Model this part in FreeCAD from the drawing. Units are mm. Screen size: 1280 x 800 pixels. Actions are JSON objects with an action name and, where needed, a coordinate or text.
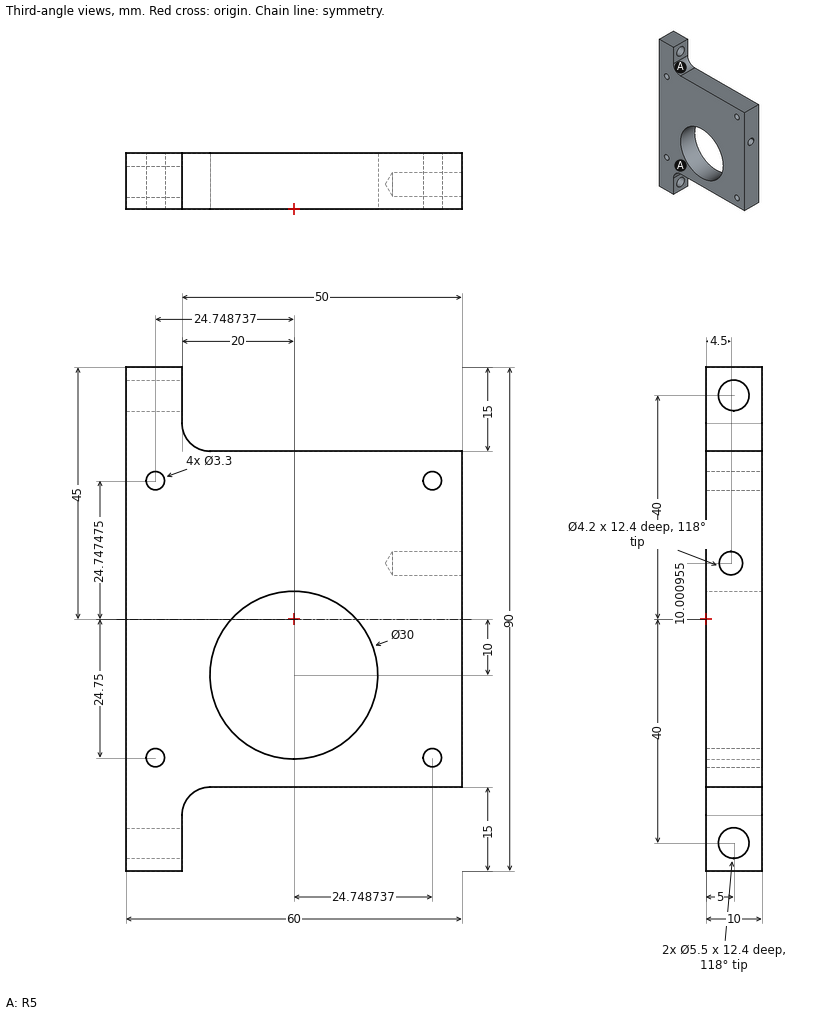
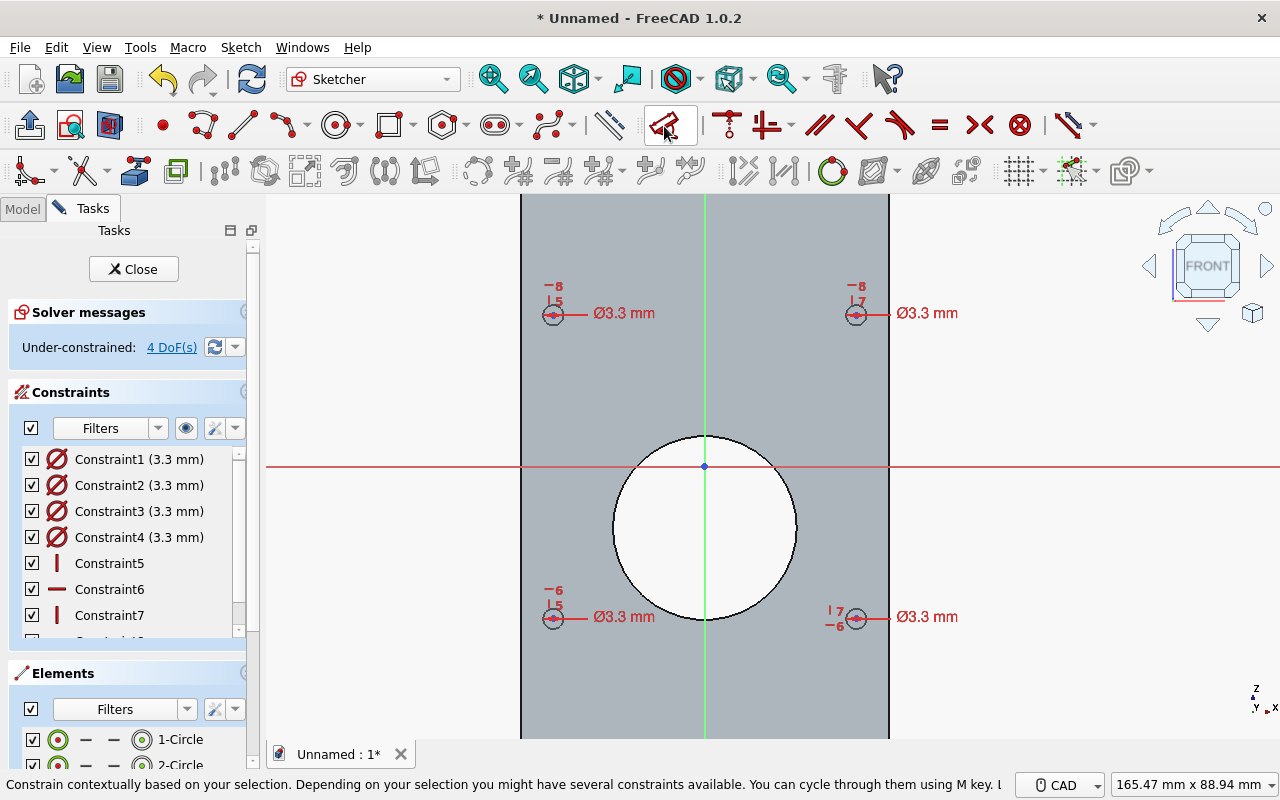
{"action": "left_click", "coordinate": [553, 619]}
{"action": "left_click", "coordinate": [519, 543]}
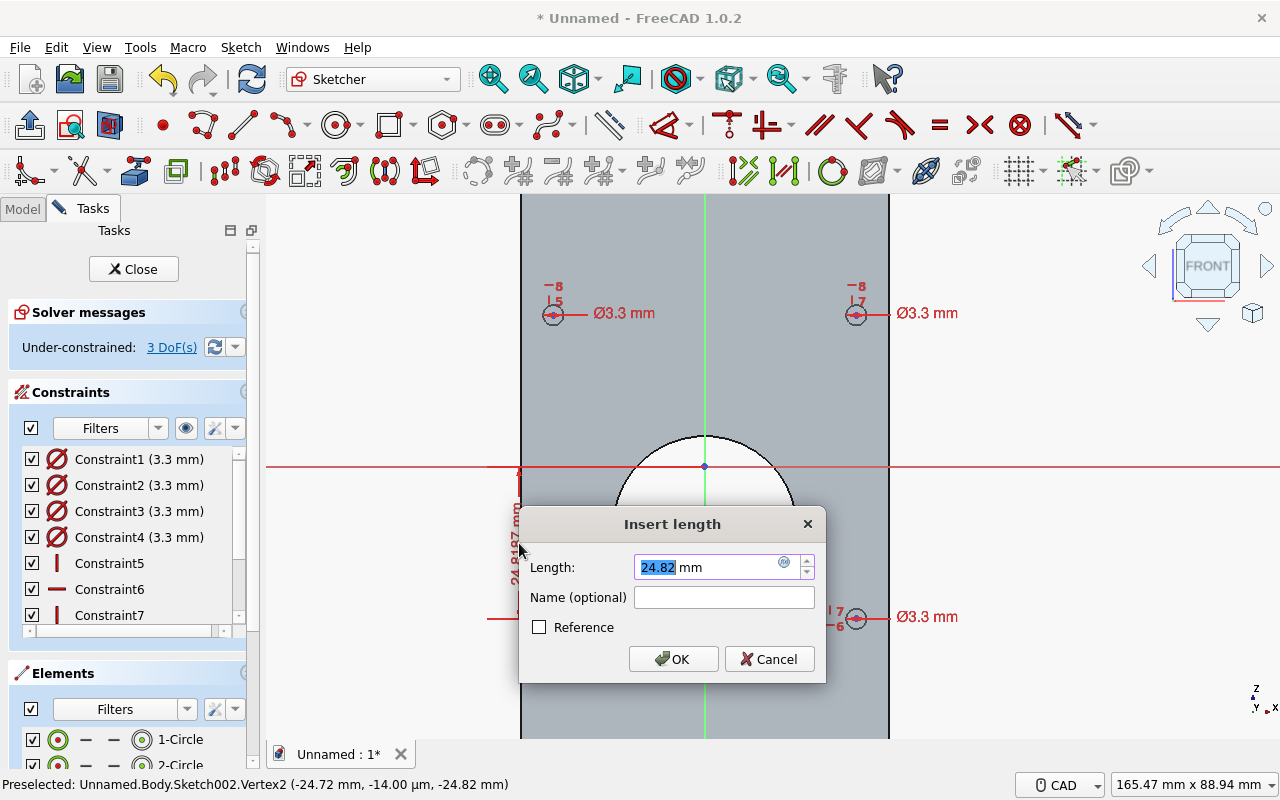
{"action": "type", "text": "24.75"}
{"action": "key", "text": "Return"}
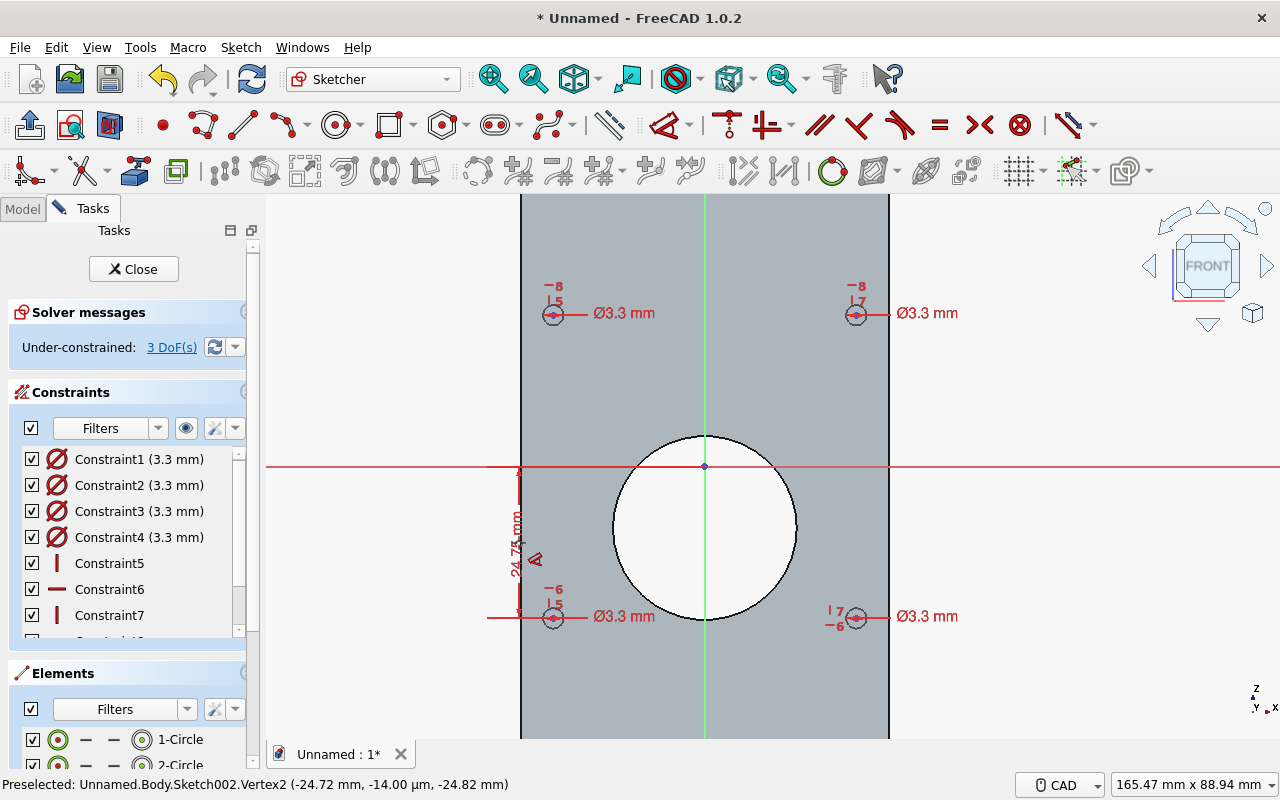
{"action": "left_click", "coordinate": [553, 315]}
{"action": "left_click", "coordinate": [629, 281]}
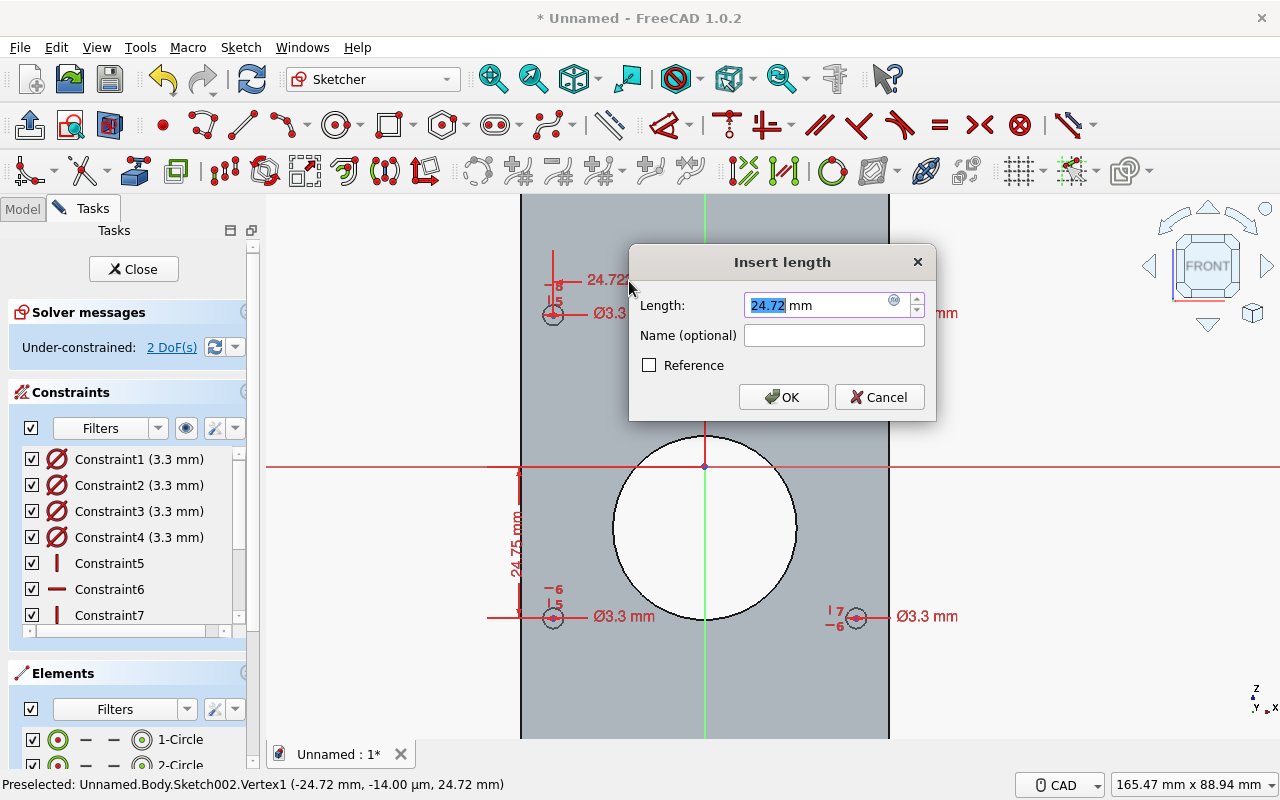
{"action": "type", "text": "24.748737"}
{"action": "key", "text": "Return"}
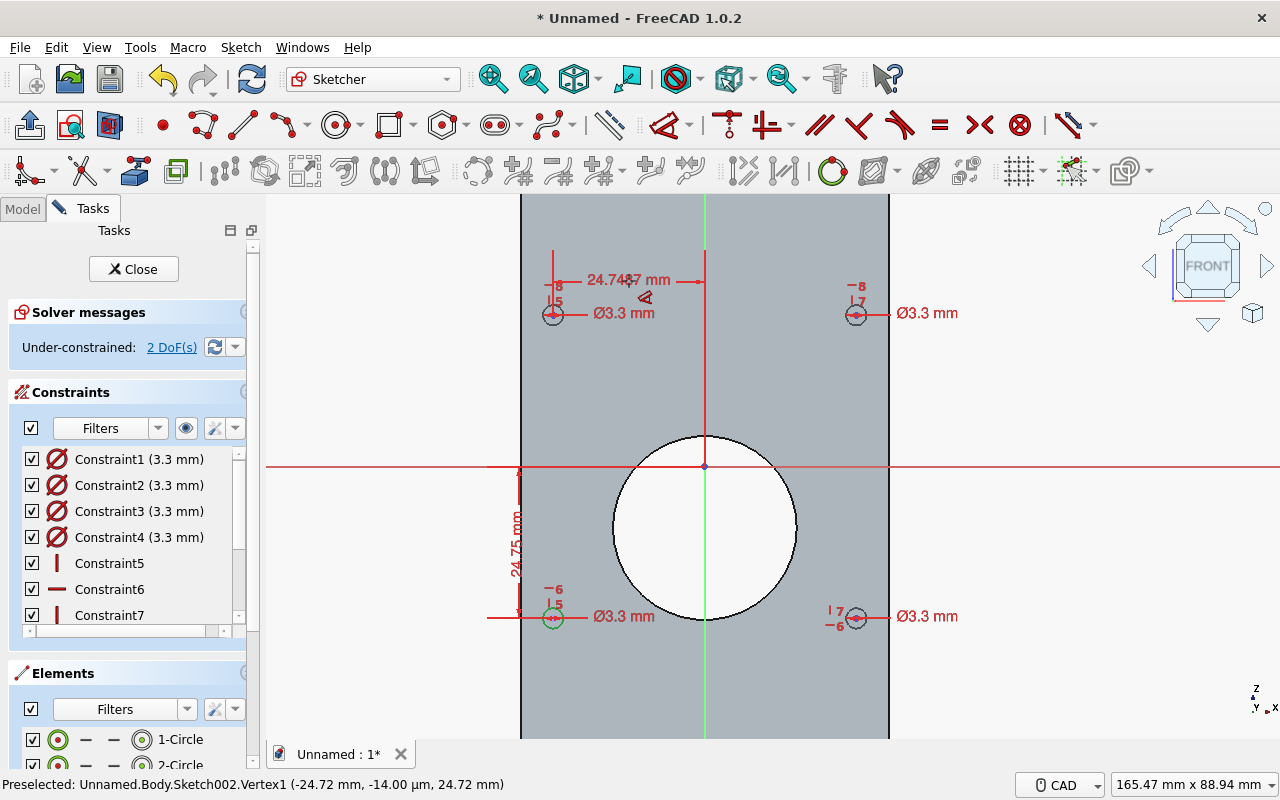
{"action": "left_click", "coordinate": [553, 315]}
{"action": "left_click", "coordinate": [519, 391]}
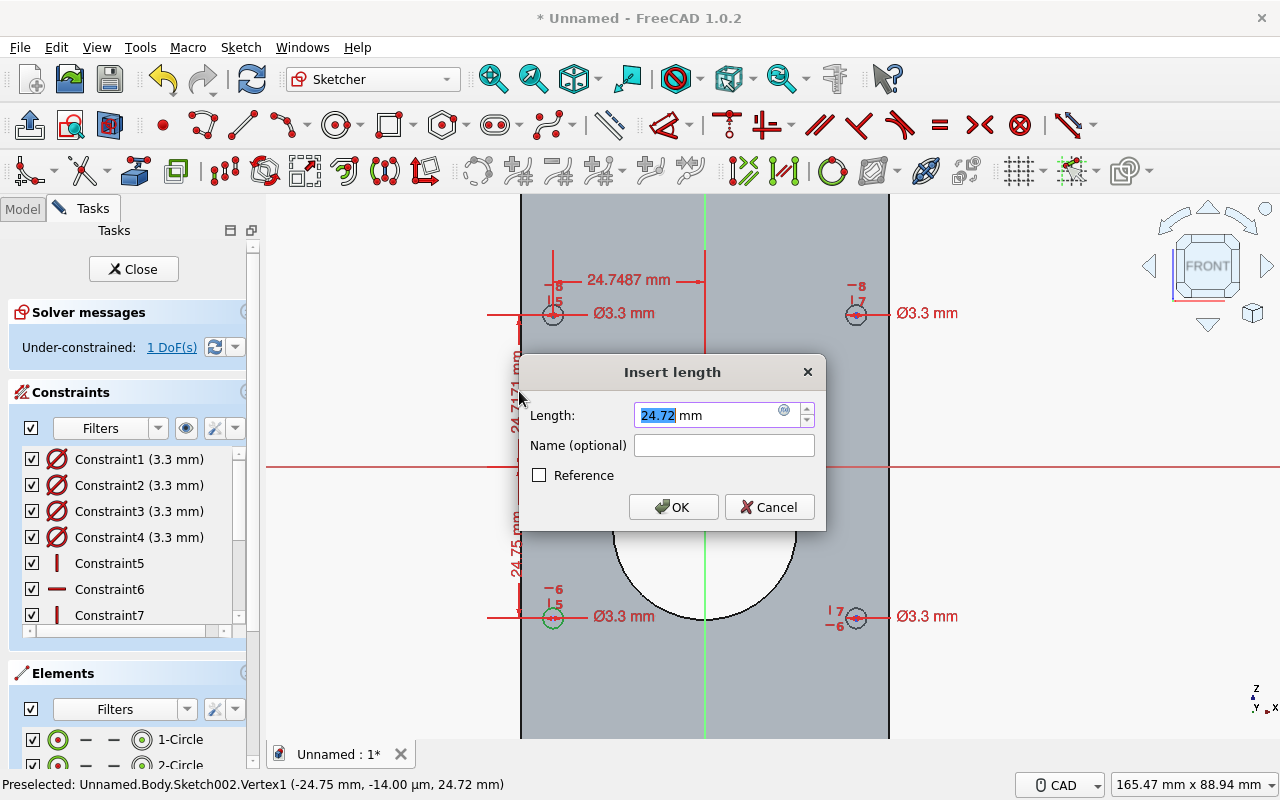
{"action": "type", "text": "24.747475"}
{"action": "key", "text": "Return"}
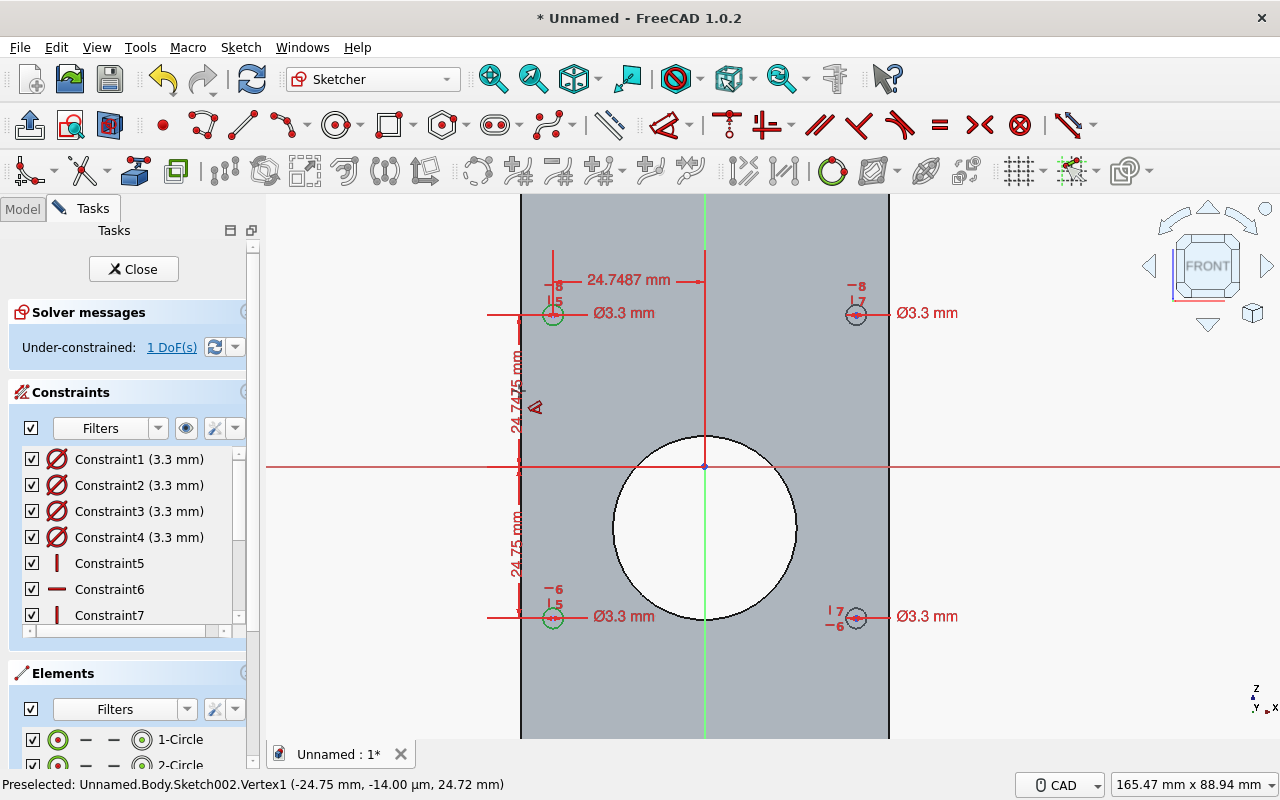
{"action": "left_click", "coordinate": [856, 618]}
{"action": "left_click", "coordinate": [781, 652]}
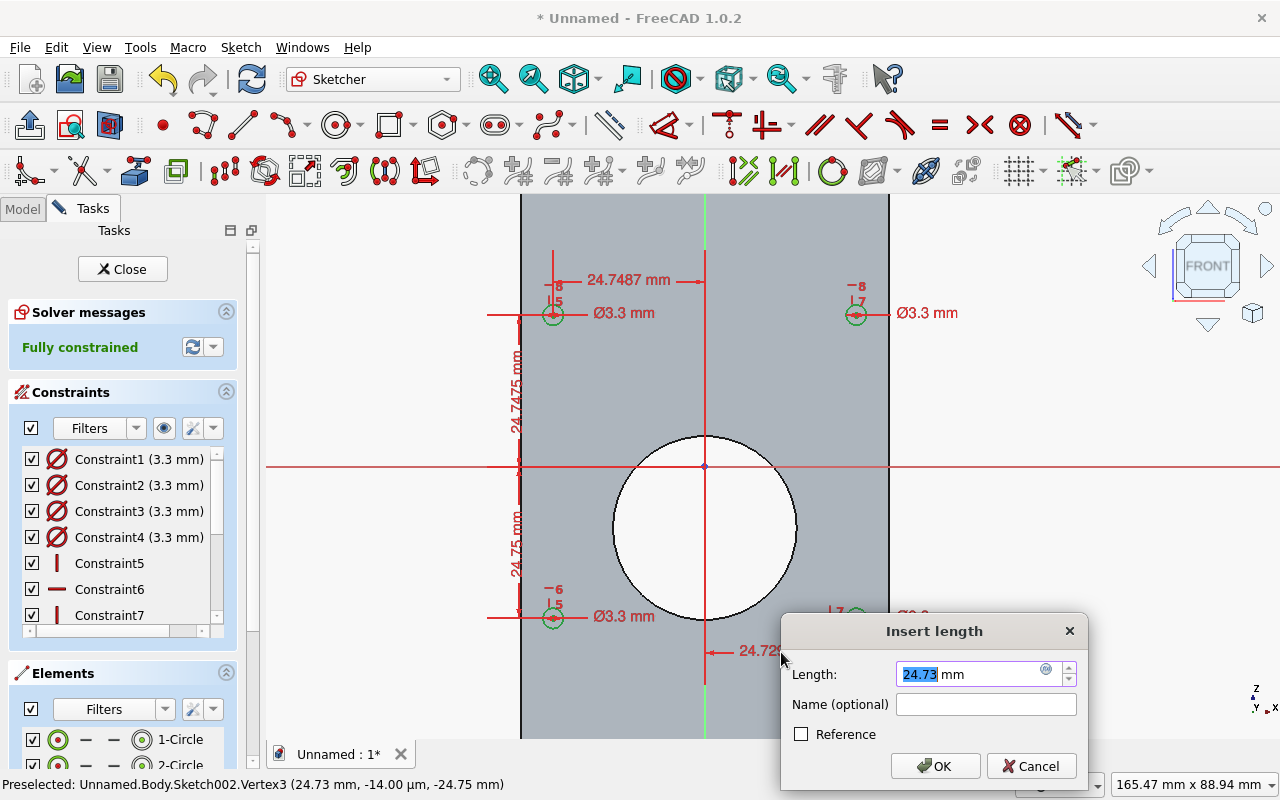
{"action": "type", "text": "24.748737"}
{"action": "key", "text": "Return"}
{"action": "key", "text": "Escape"}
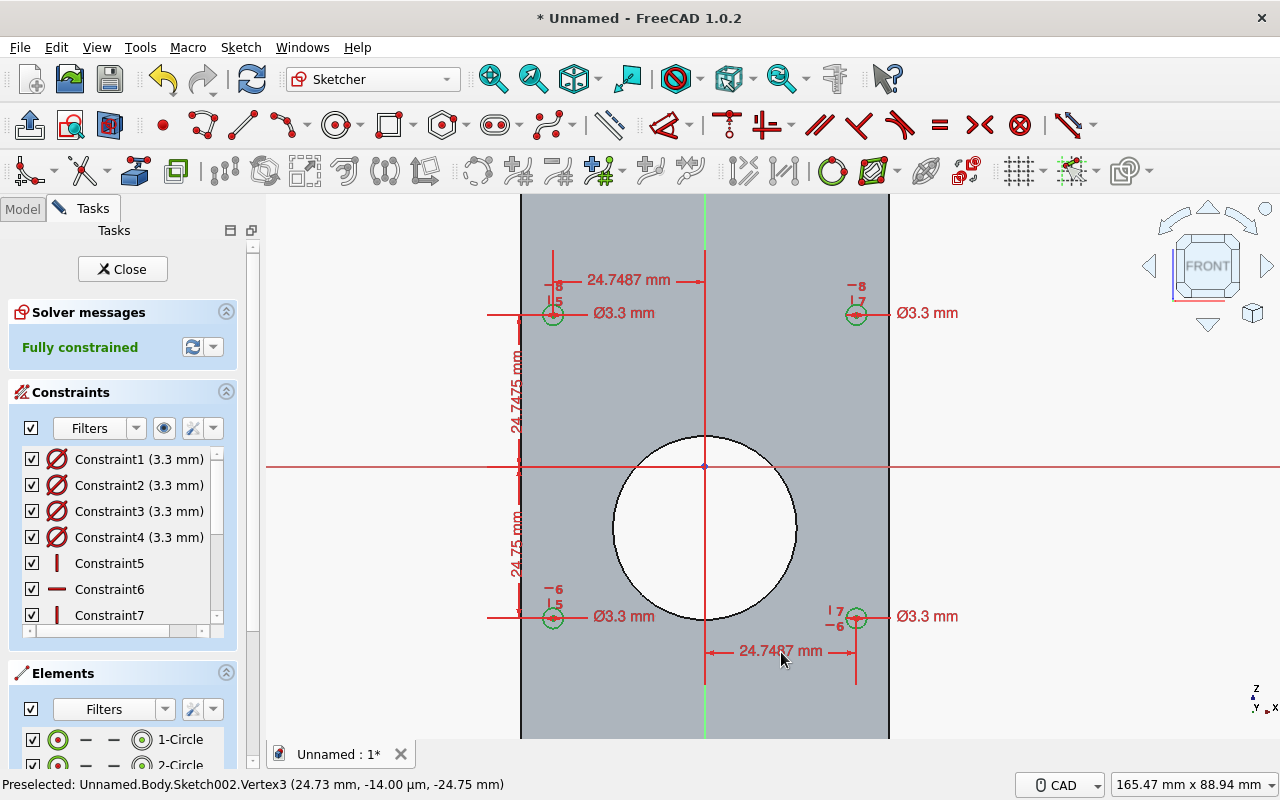
{"action": "left_click", "coordinate": [123, 269]}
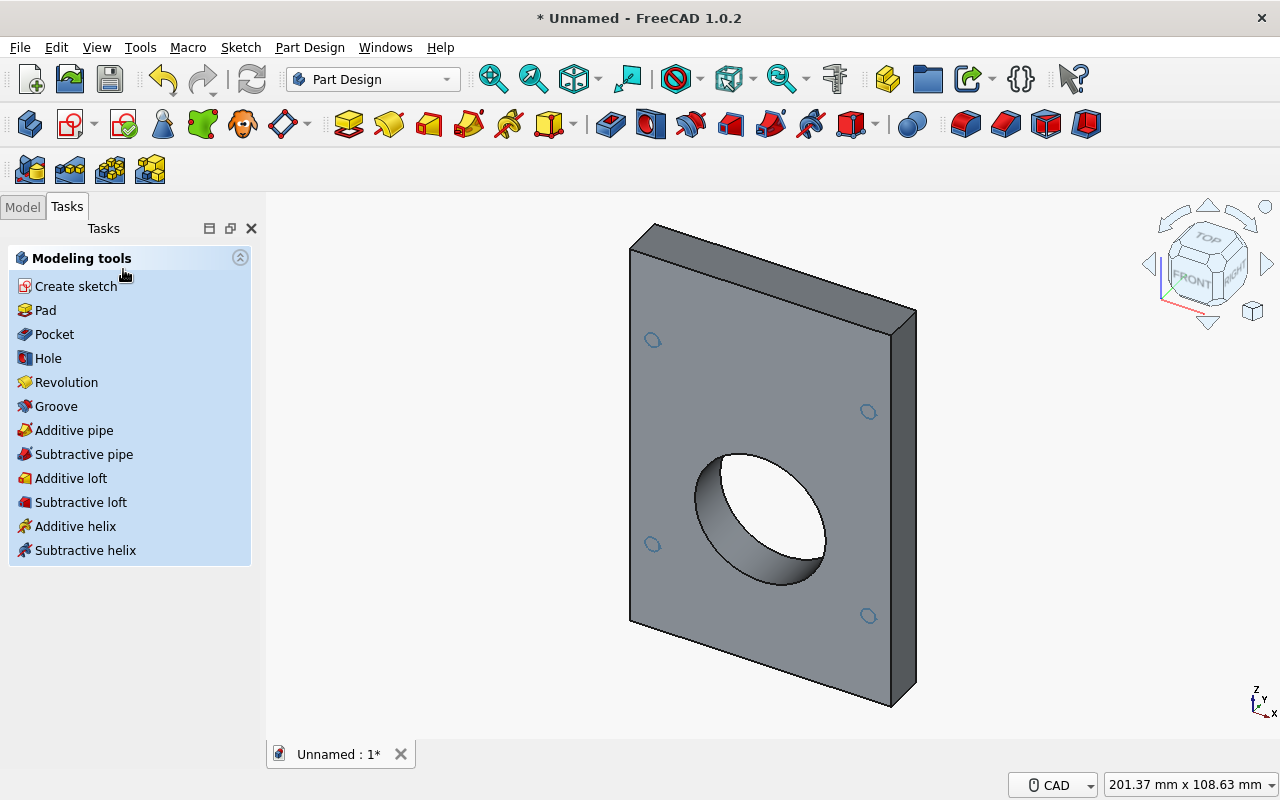
{"action": "left_click", "coordinate": [612, 124]}